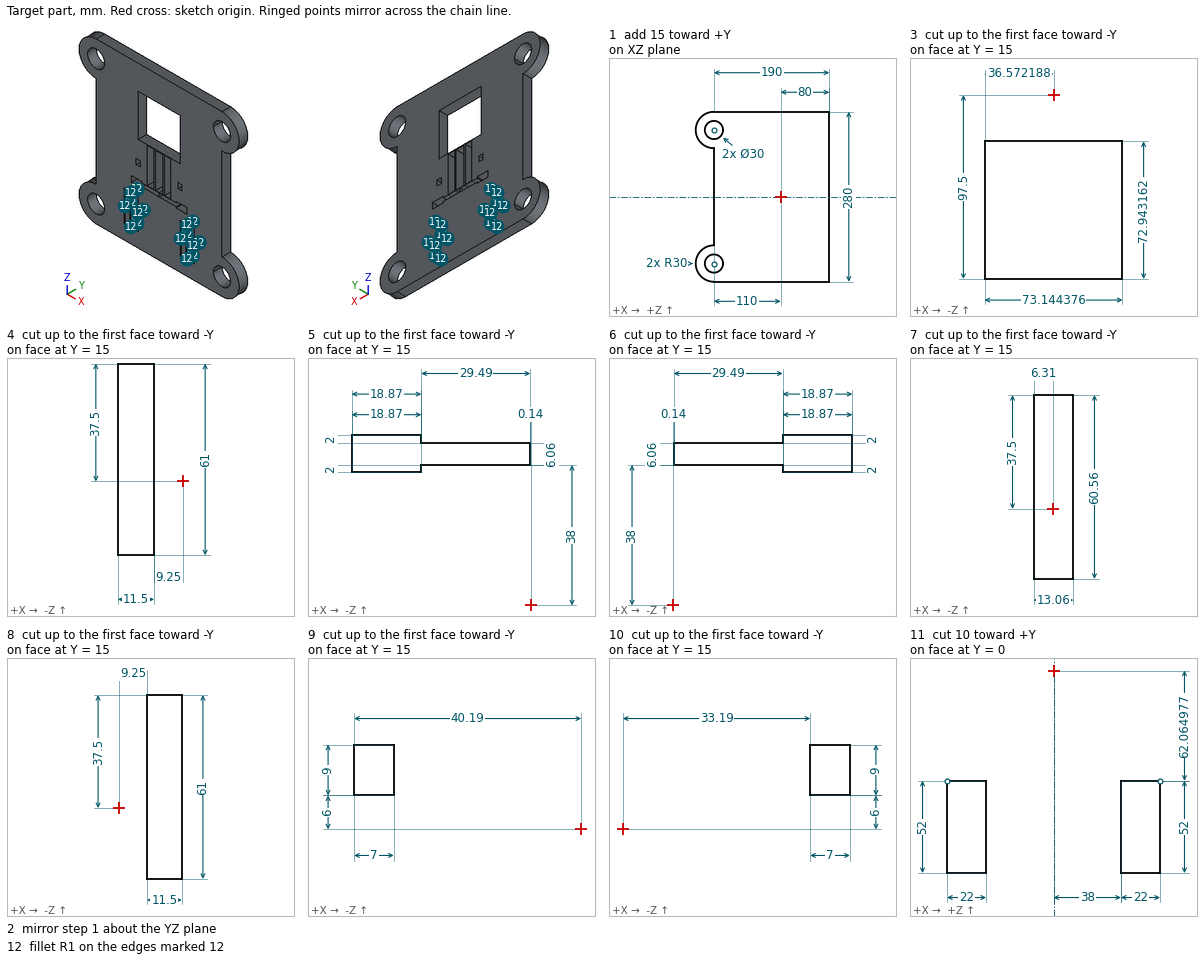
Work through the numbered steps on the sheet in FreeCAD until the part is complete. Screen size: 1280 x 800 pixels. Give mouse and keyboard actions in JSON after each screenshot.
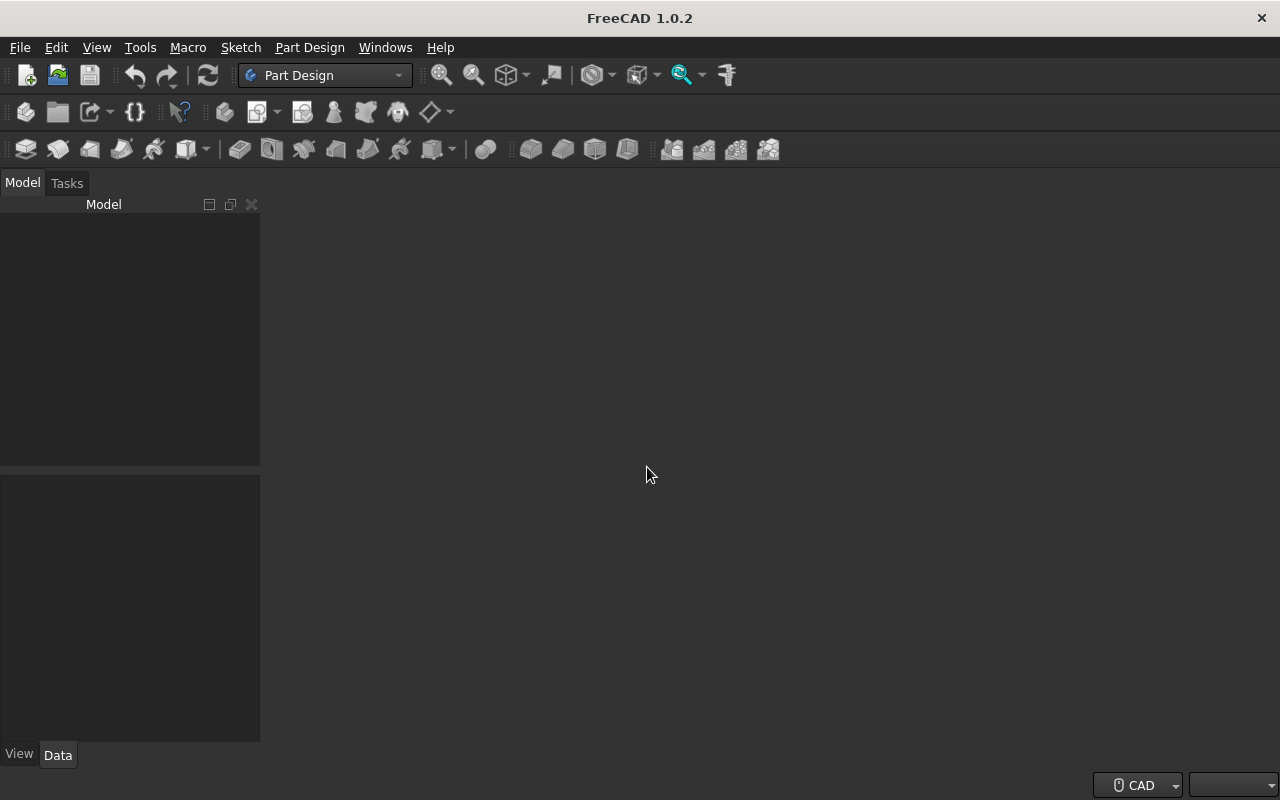
{"action": "left_click", "coordinate": [26, 76]}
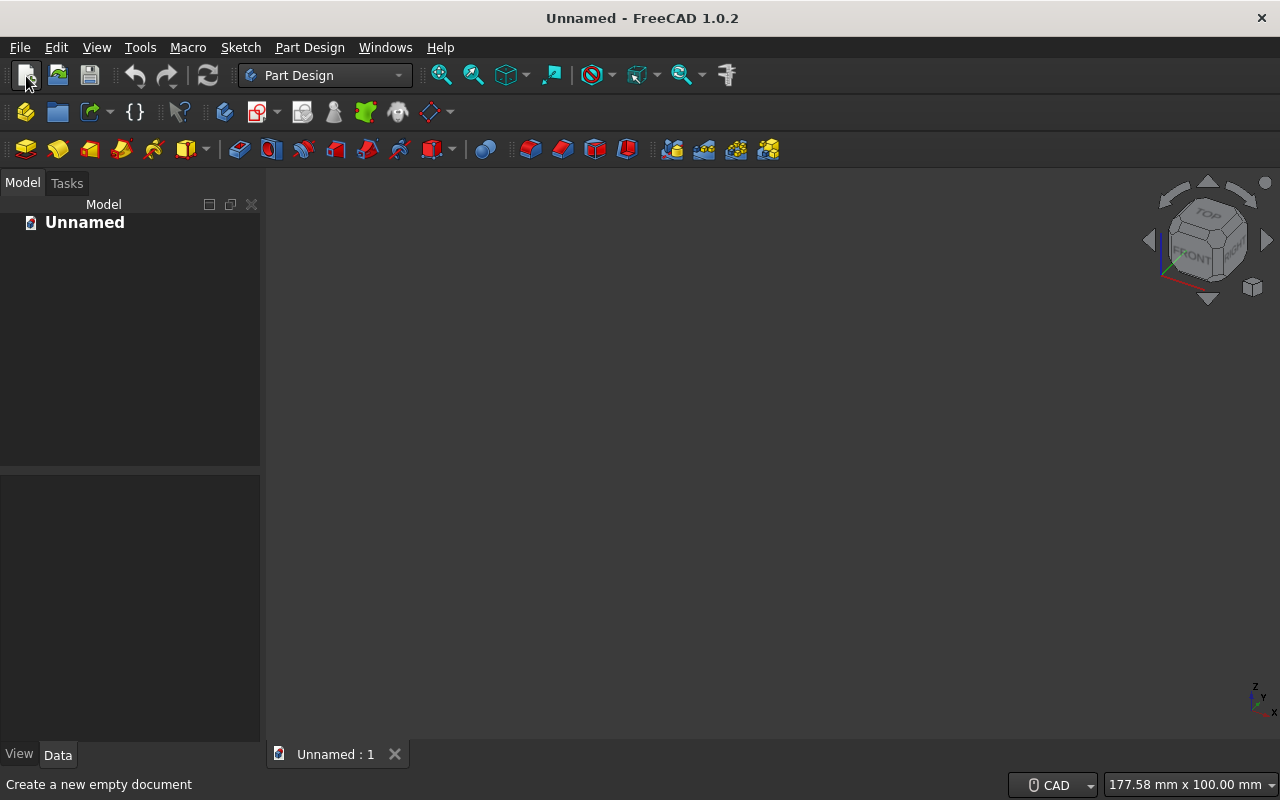
{"action": "left_click", "coordinate": [258, 112]}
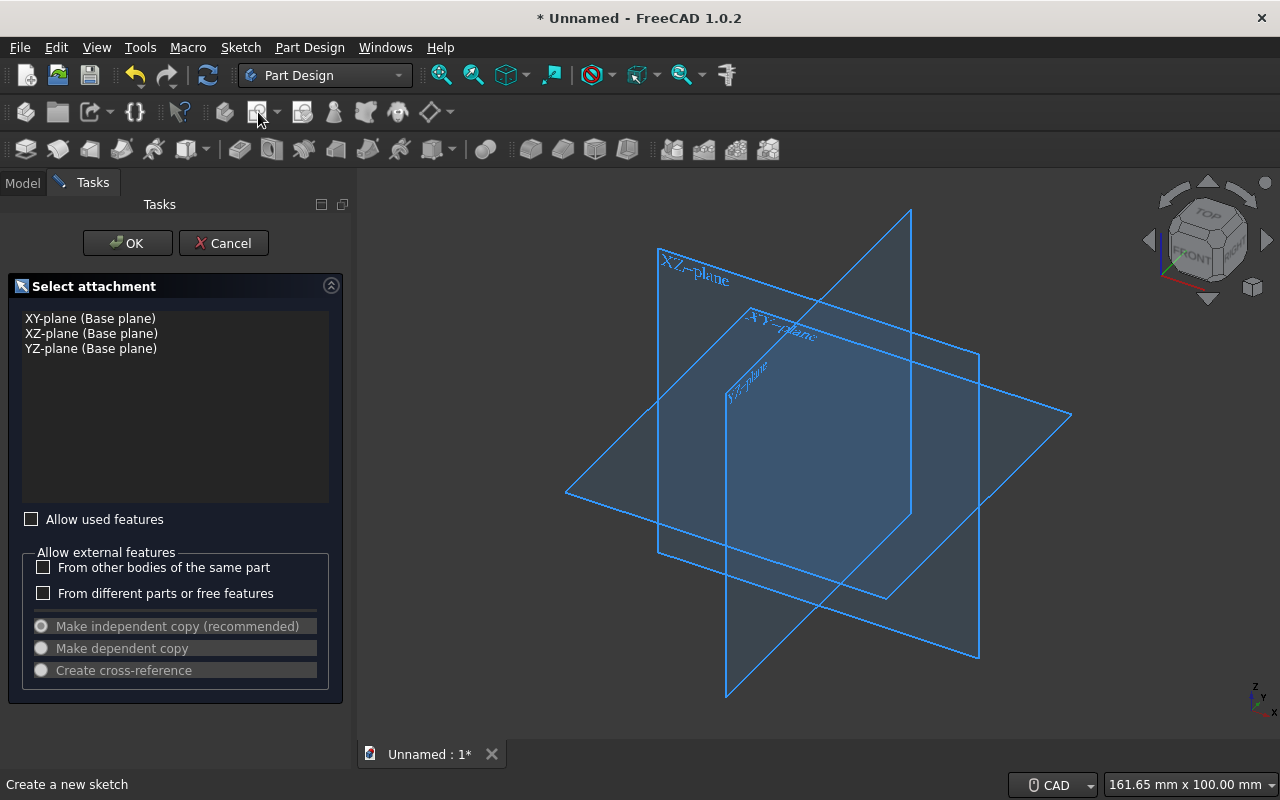
{"action": "left_click", "coordinate": [82, 334]}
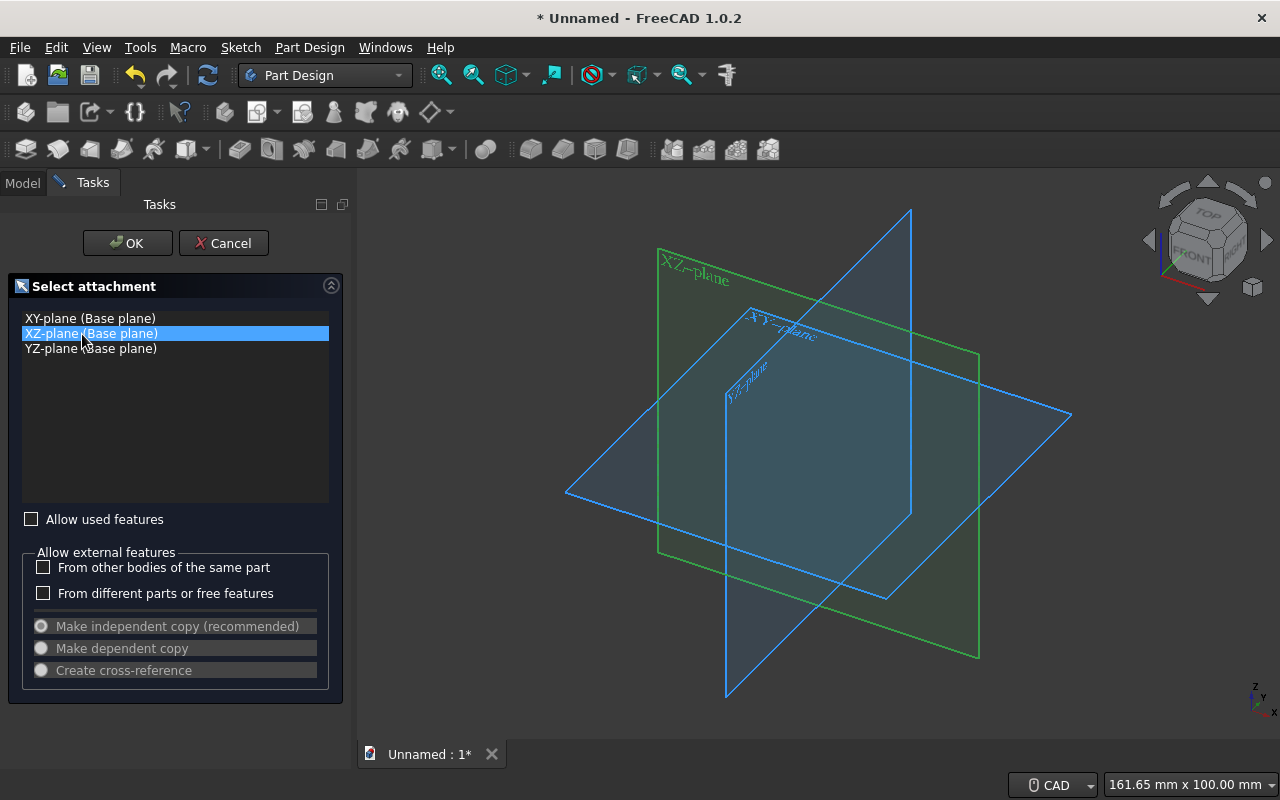
{"action": "left_click", "coordinate": [128, 243]}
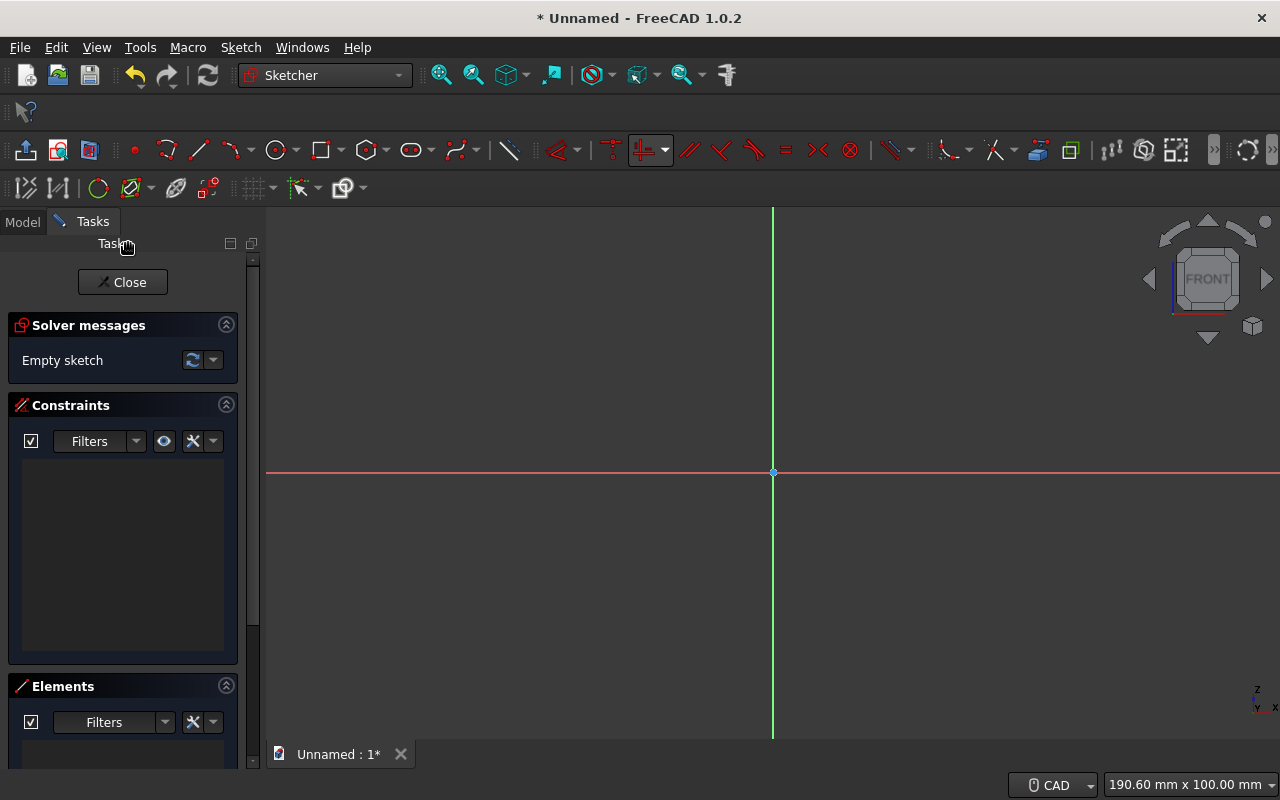
{"action": "scroll", "coordinate": [734, 473], "scroll_direction": "down", "scroll_amount": 7}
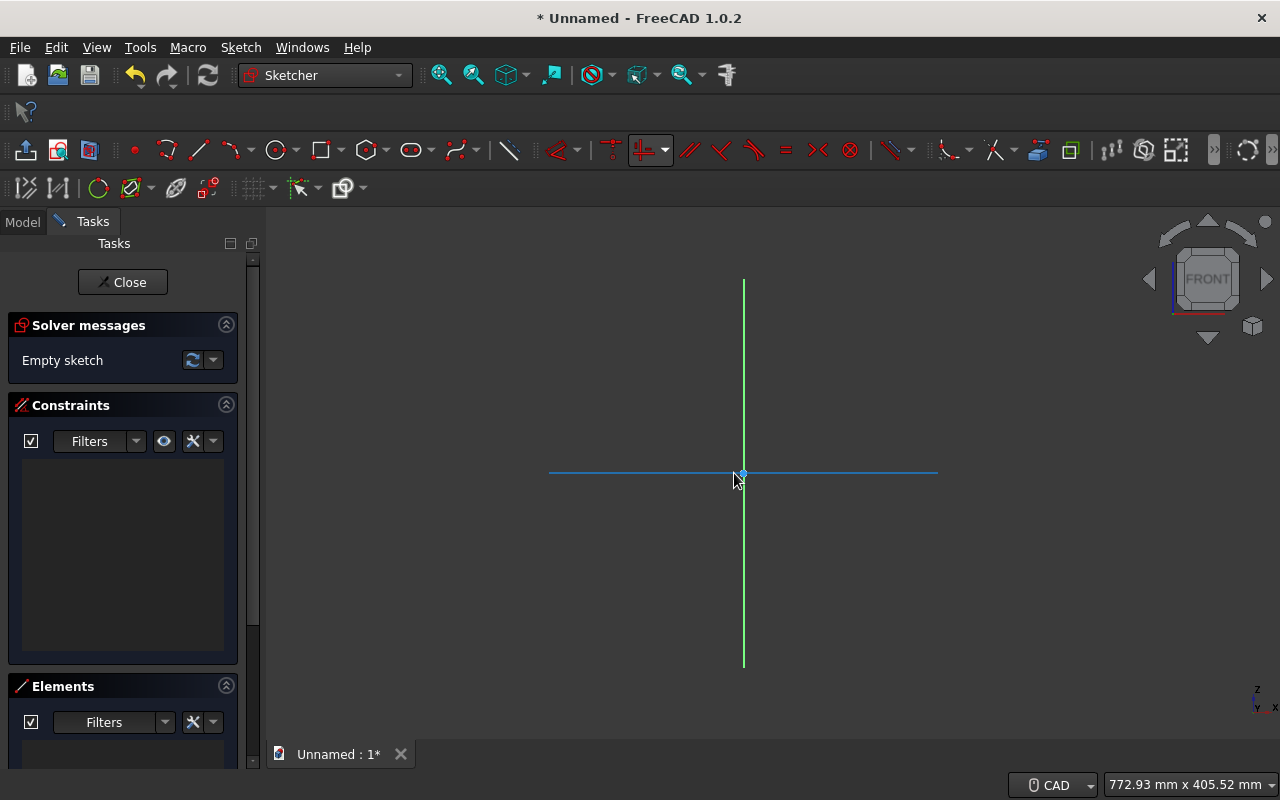
{"action": "left_click", "coordinate": [168, 150]}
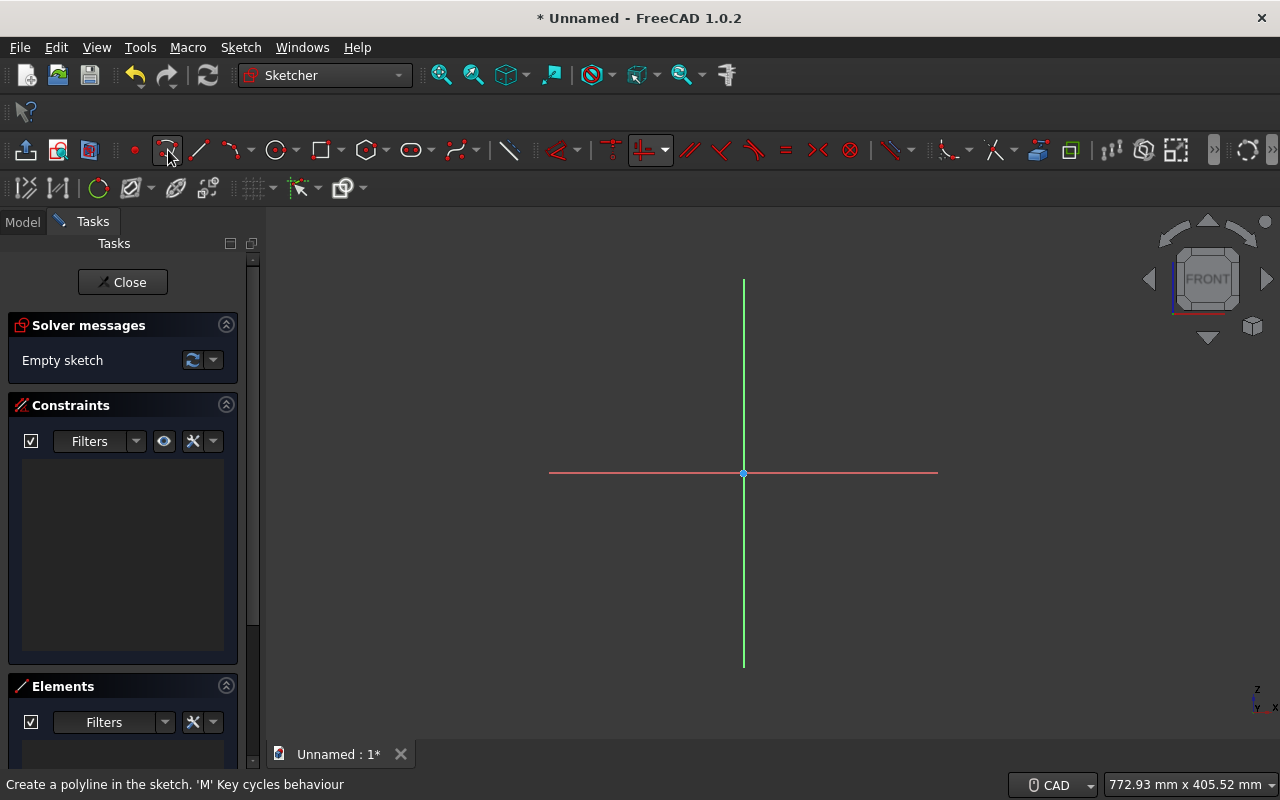
{"action": "left_click", "coordinate": [600, 290]}
{"action": "left_click", "coordinate": [849, 290]}
{"action": "left_click", "coordinate": [849, 657]}
{"action": "left_click", "coordinate": [600, 657]}
{"action": "right_click", "coordinate": [600, 657]}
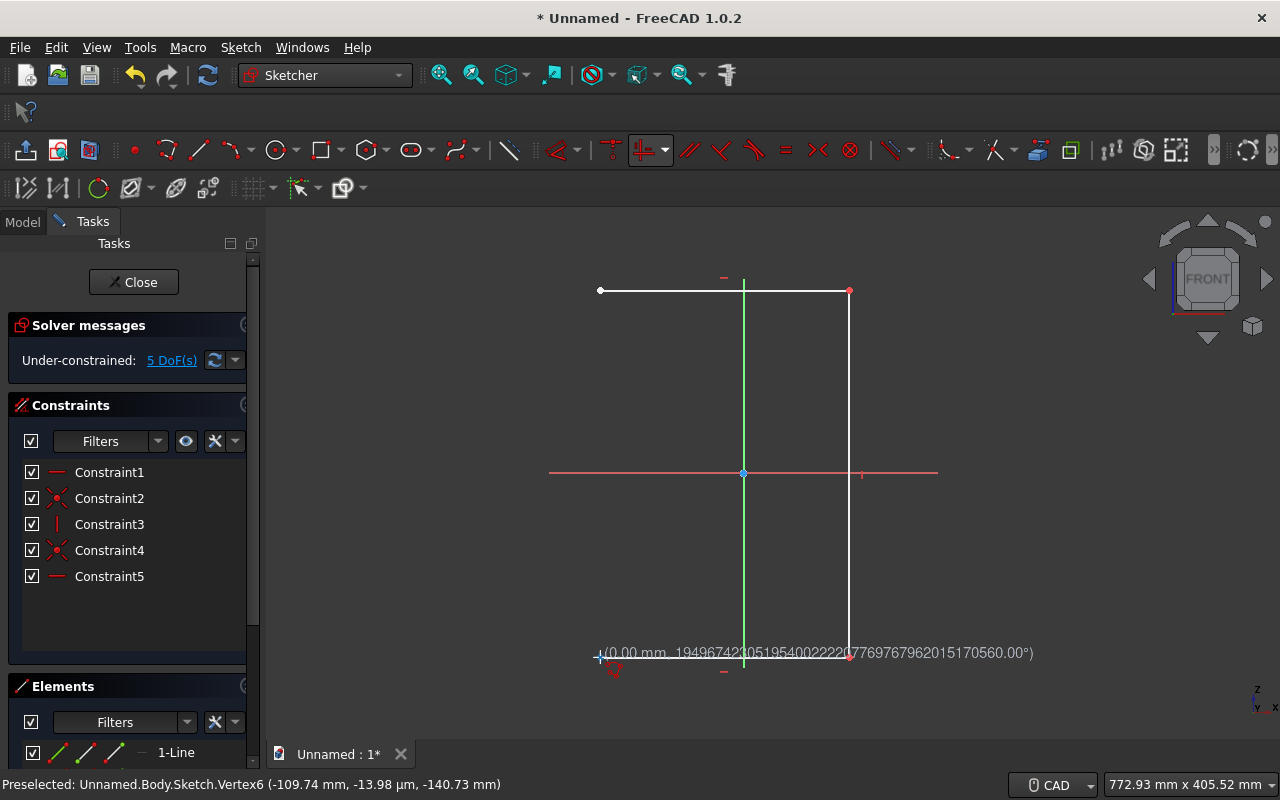
{"action": "left_click", "coordinate": [200, 150]}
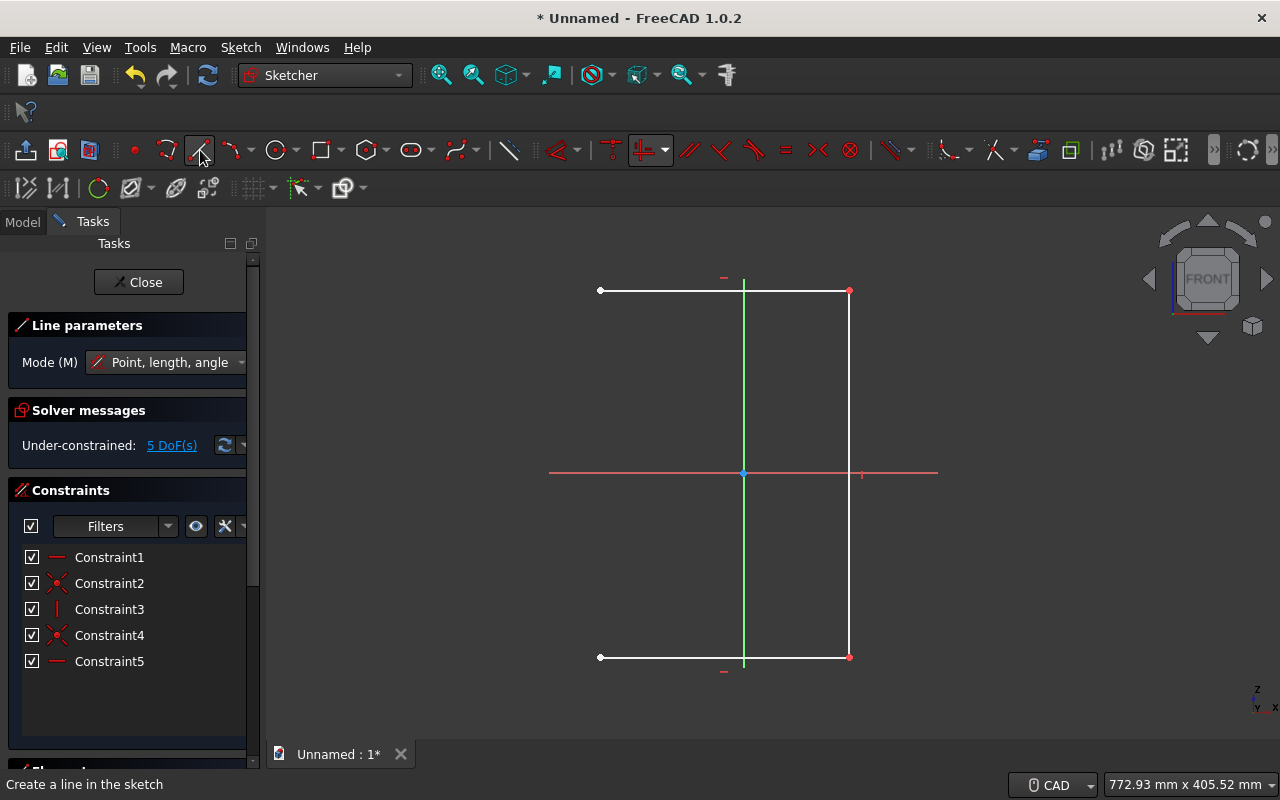
{"action": "left_click", "coordinate": [600, 578]}
{"action": "left_click", "coordinate": [600, 368]}